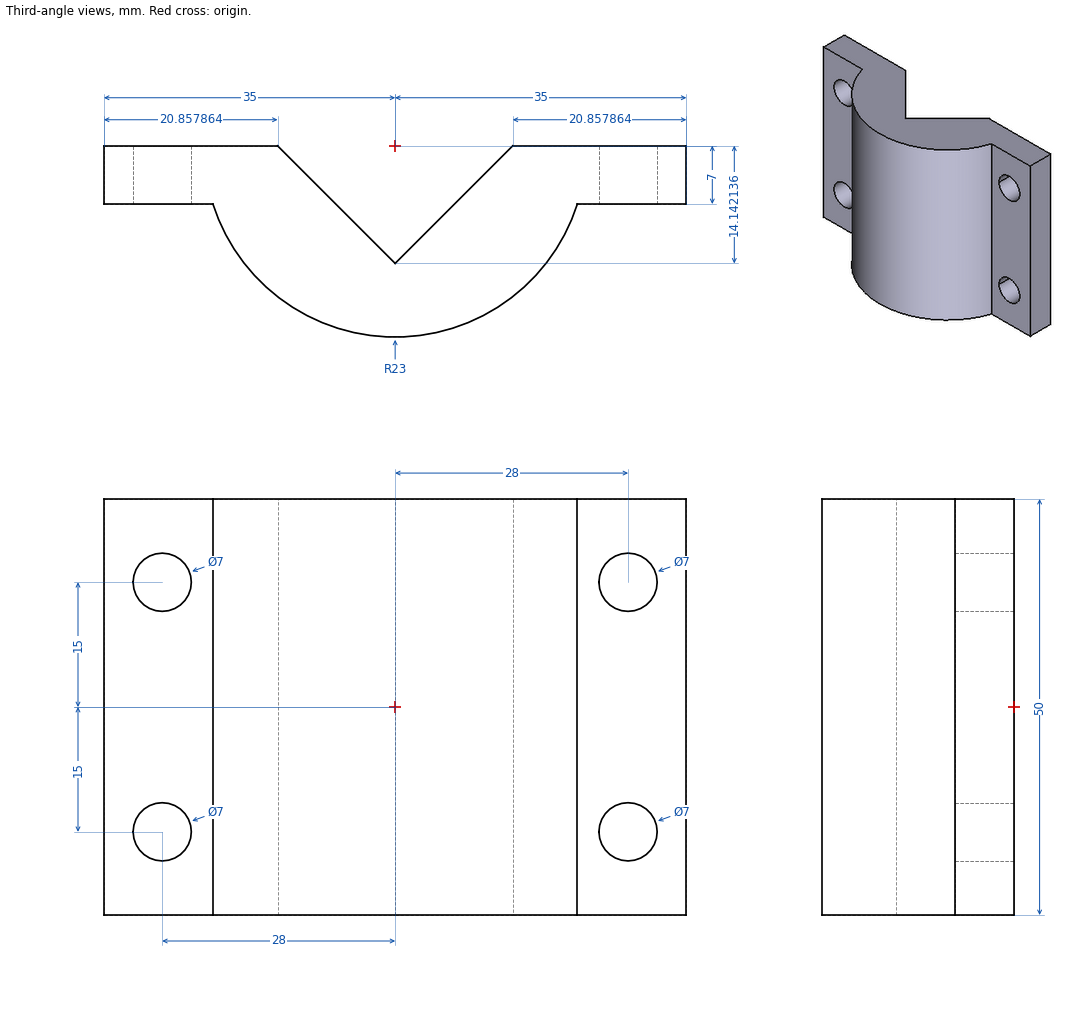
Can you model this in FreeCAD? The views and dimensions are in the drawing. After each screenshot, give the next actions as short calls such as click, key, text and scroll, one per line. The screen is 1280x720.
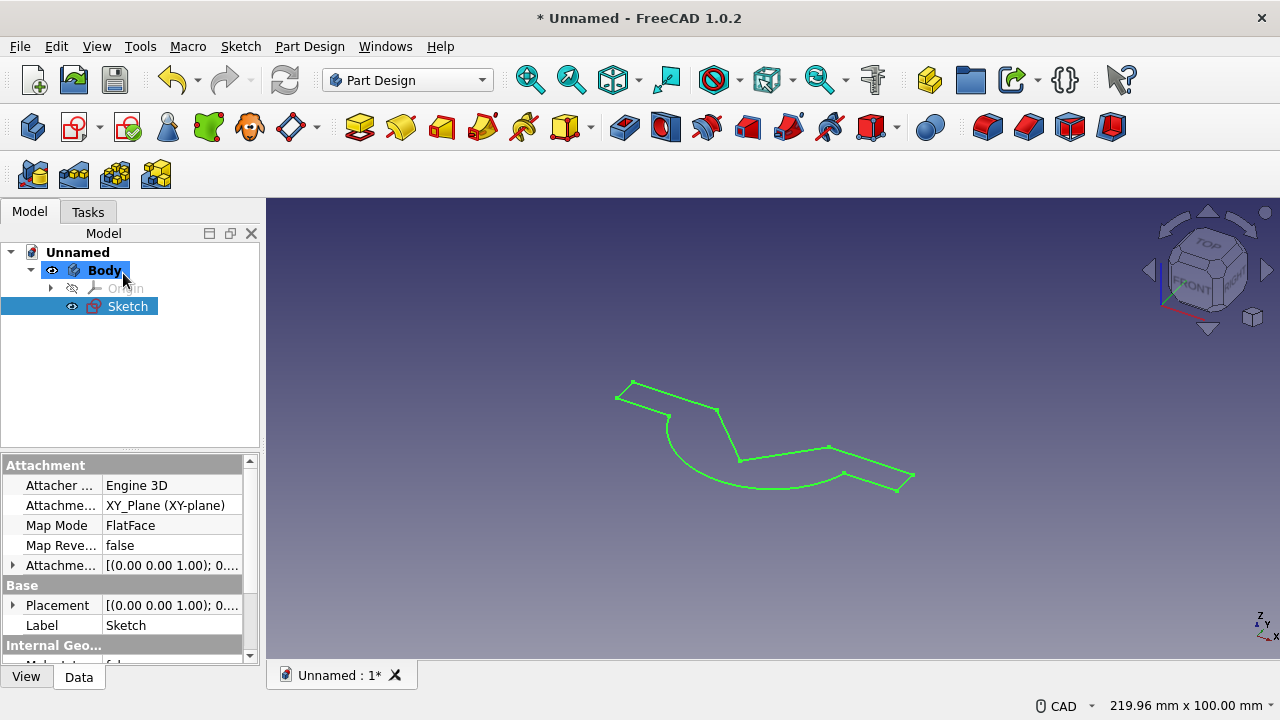
click(360, 128)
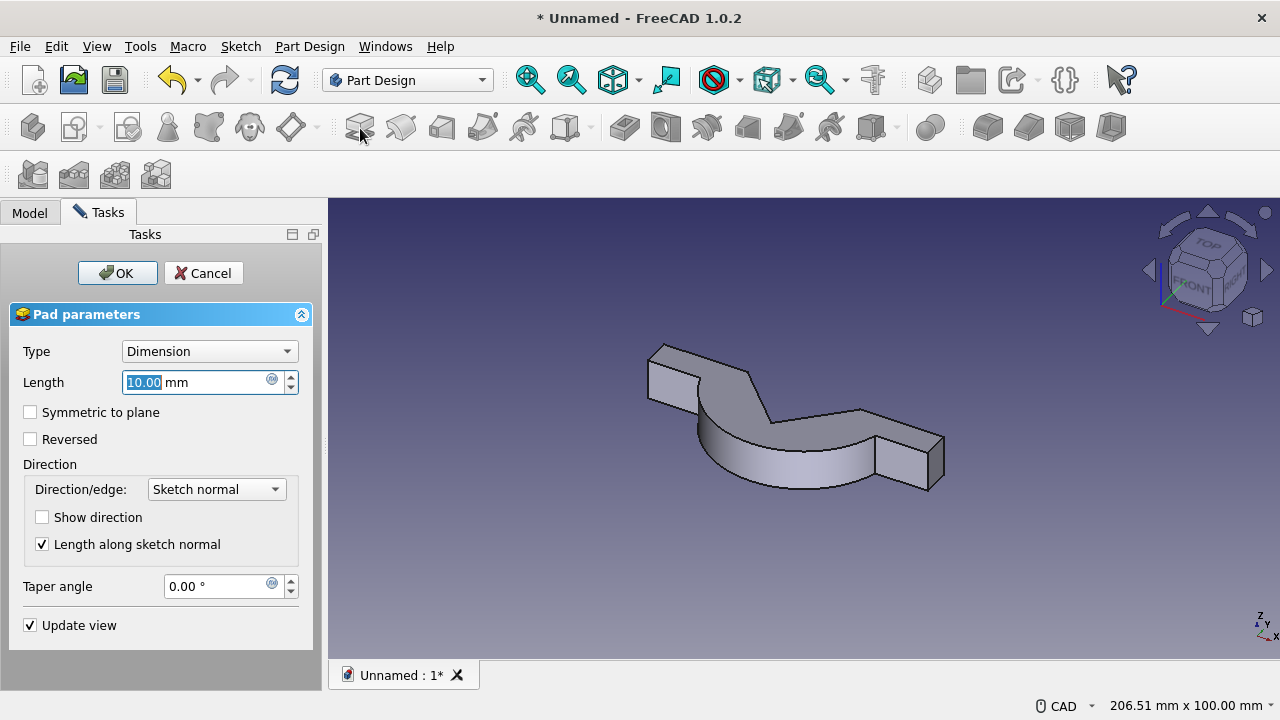
text(50)
key(Tab)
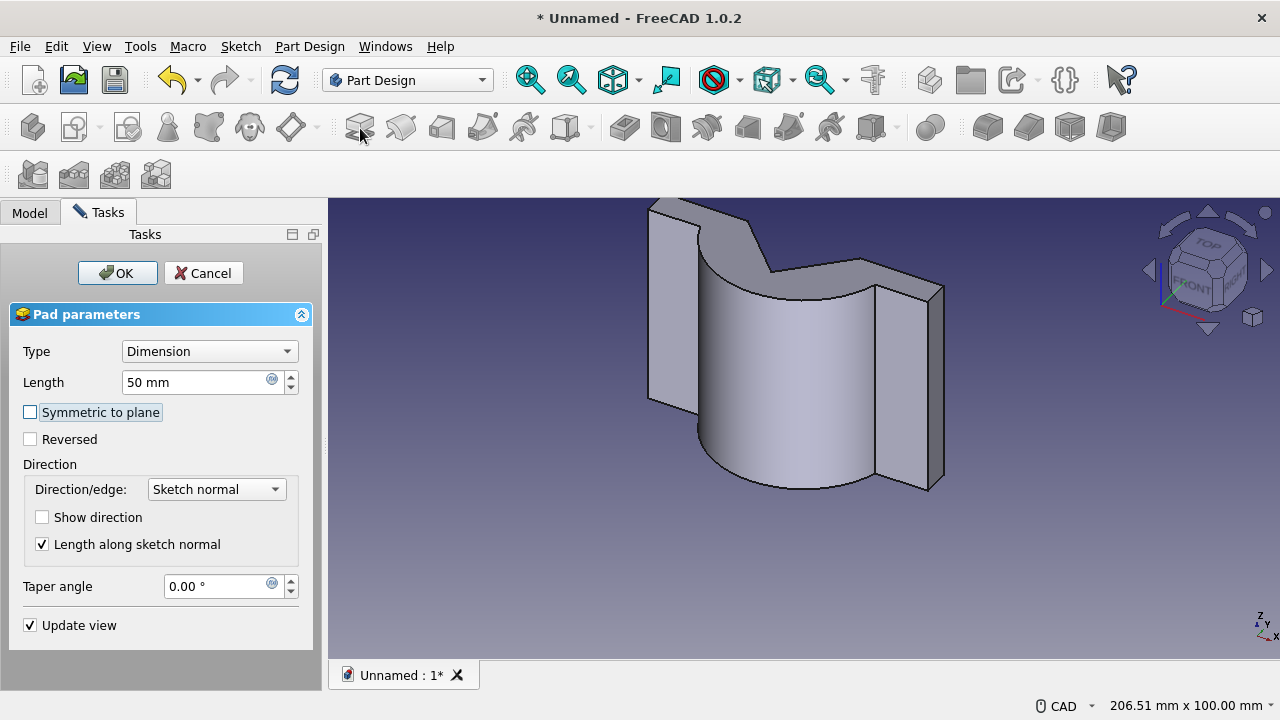
click(31, 412)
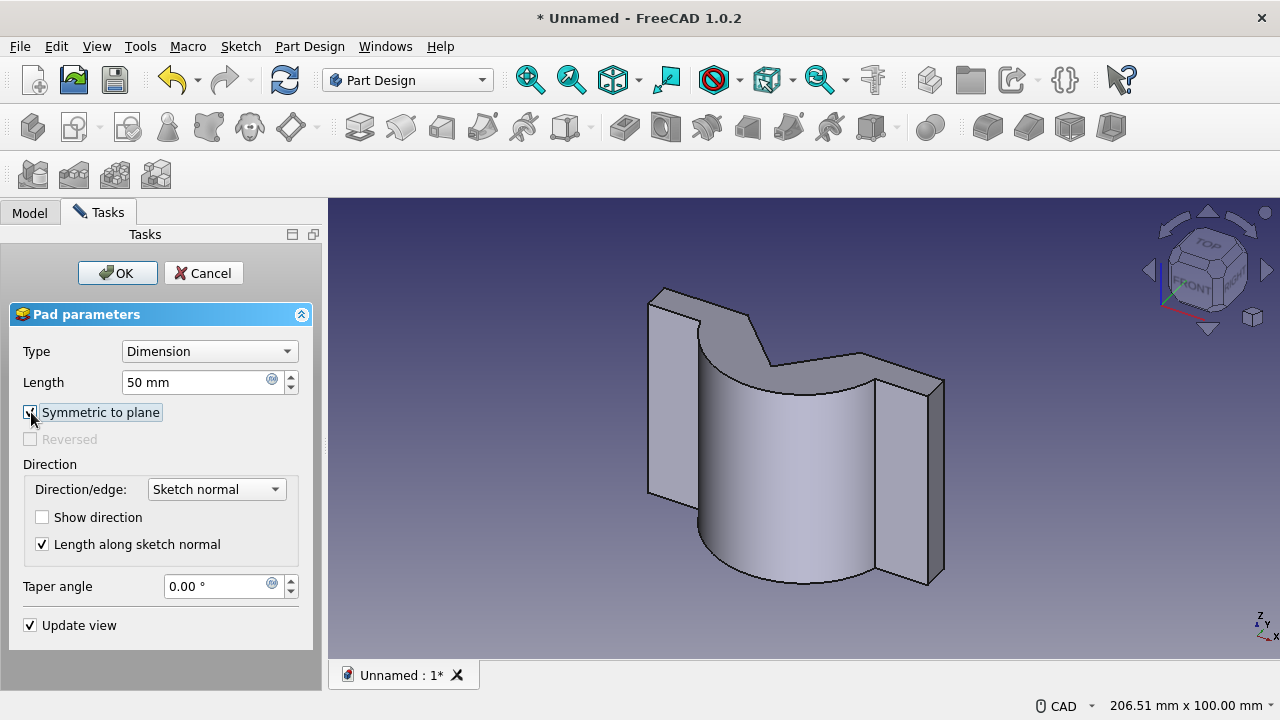
click(118, 273)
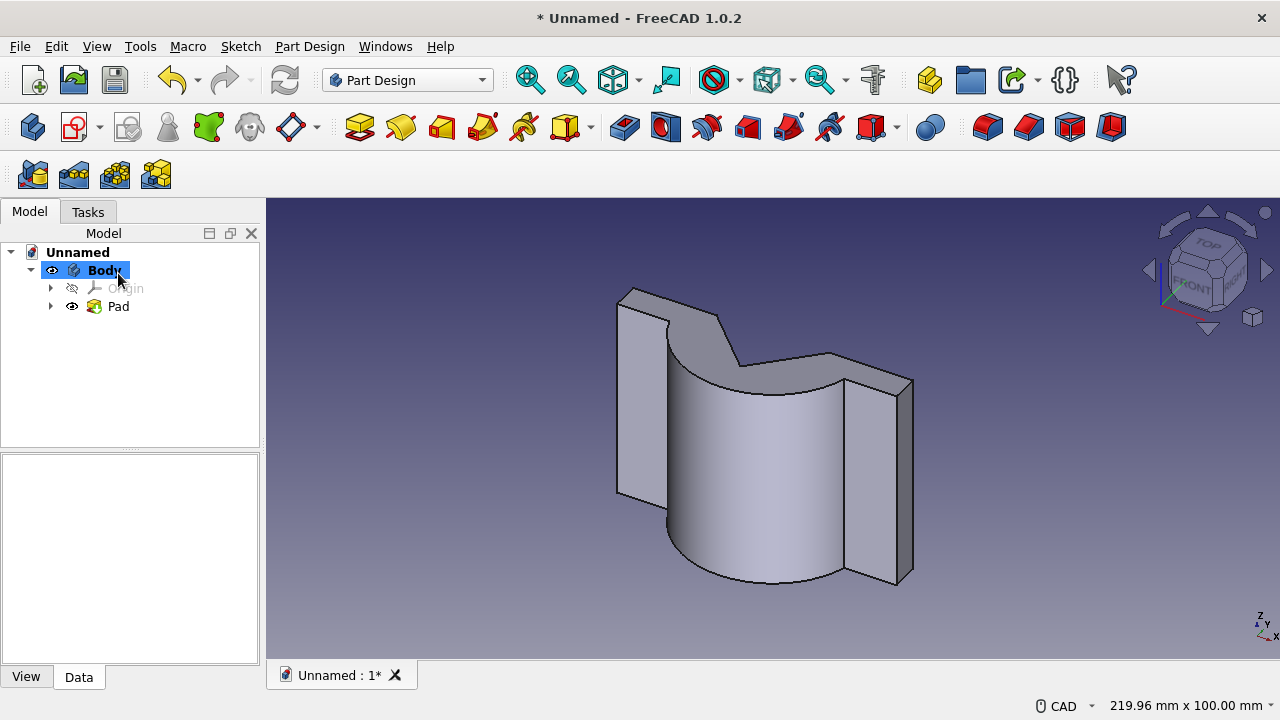
click(74, 128)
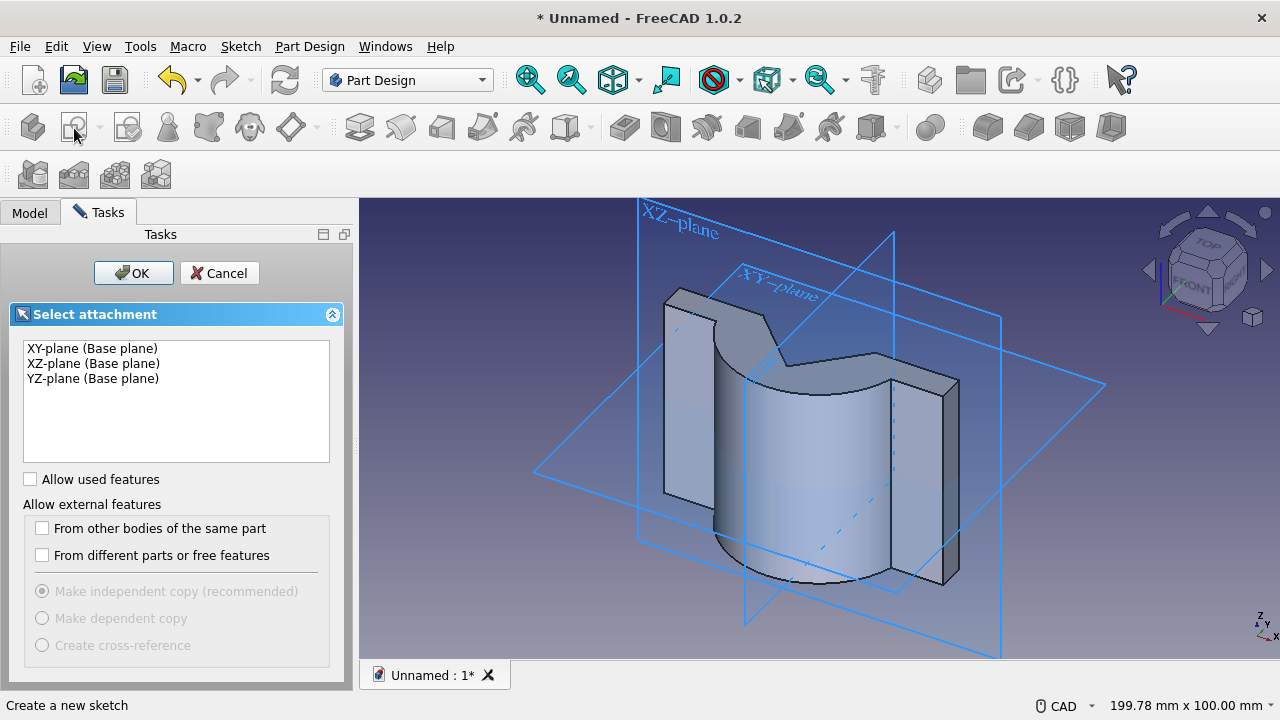
click(84, 364)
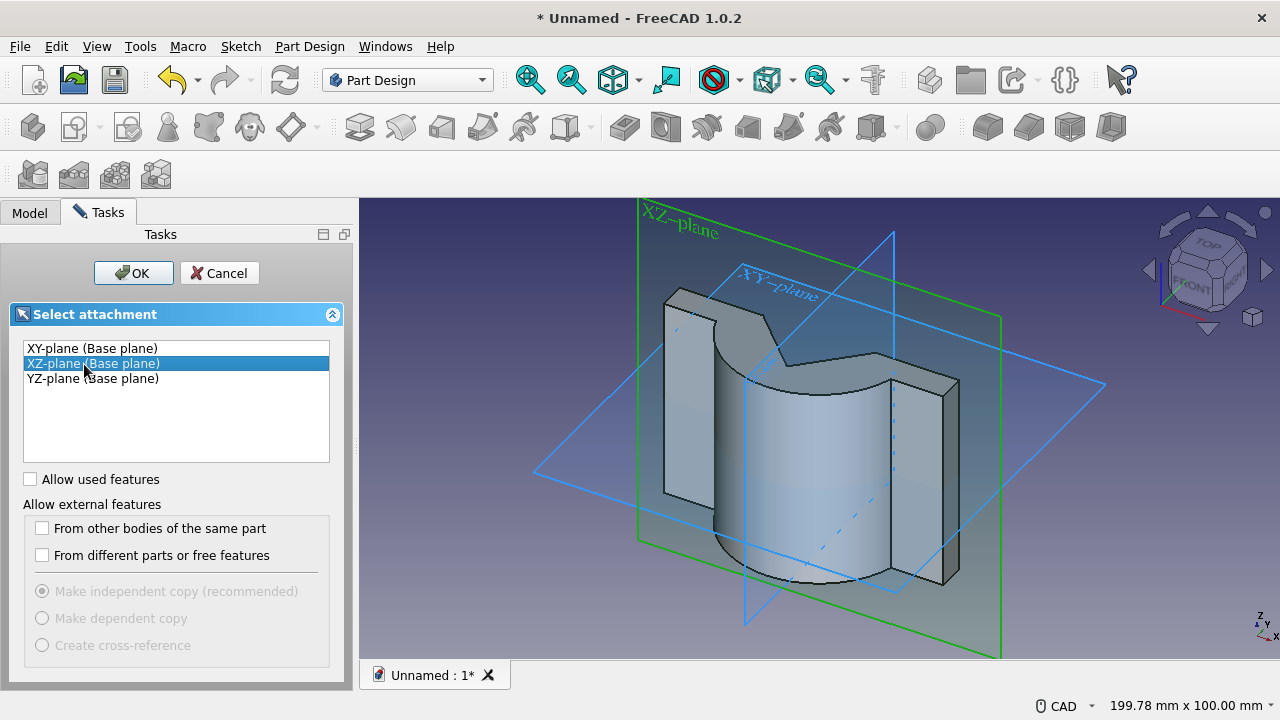
click(134, 273)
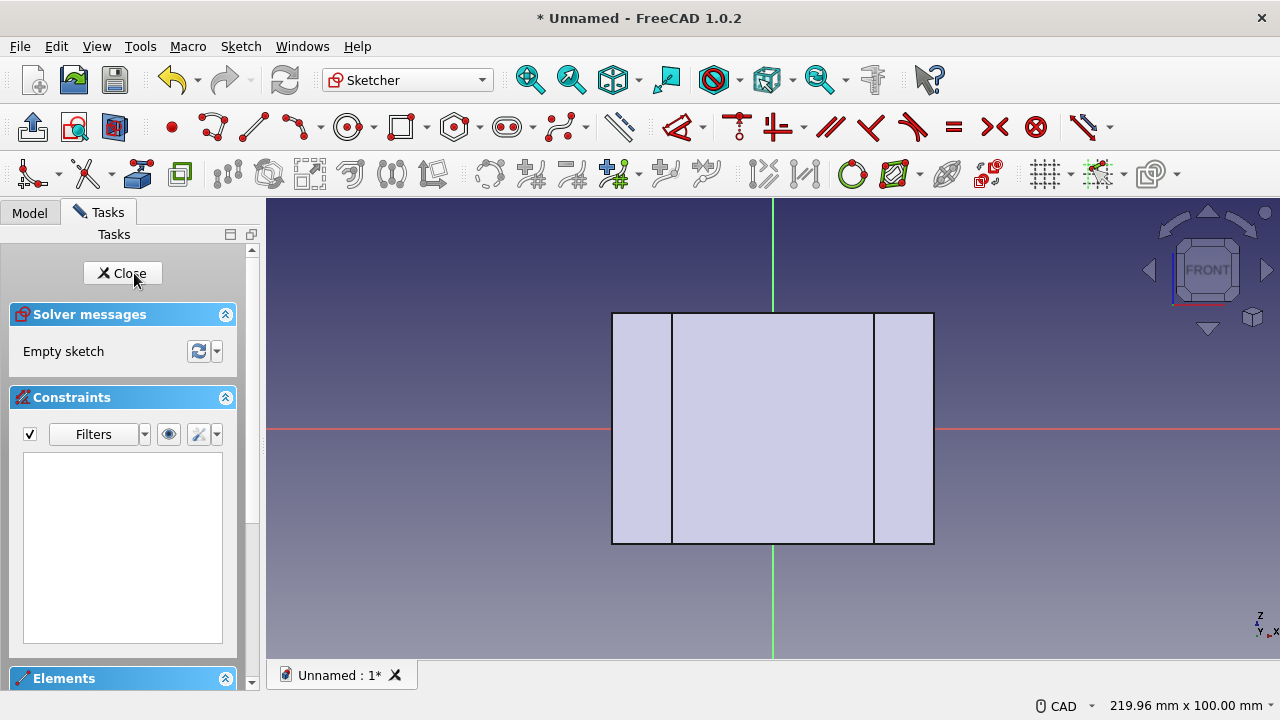
key(q)
key(s)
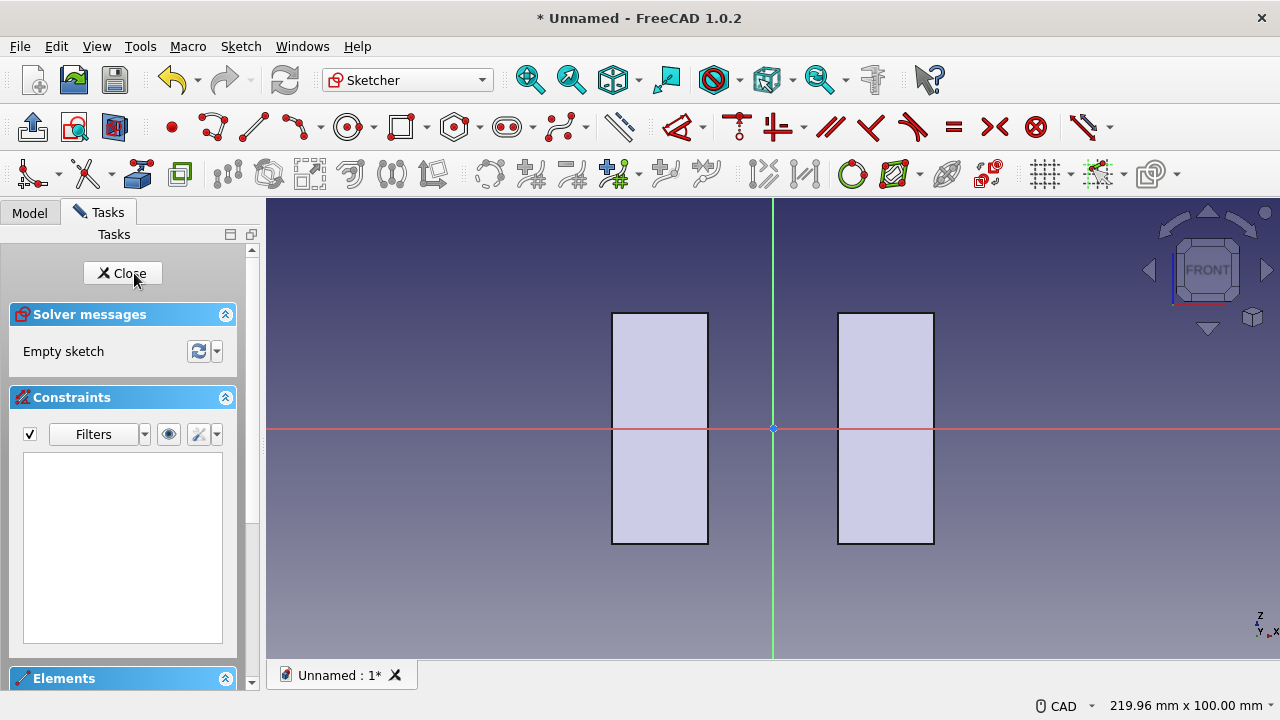
scroll(636, 506, up, 11)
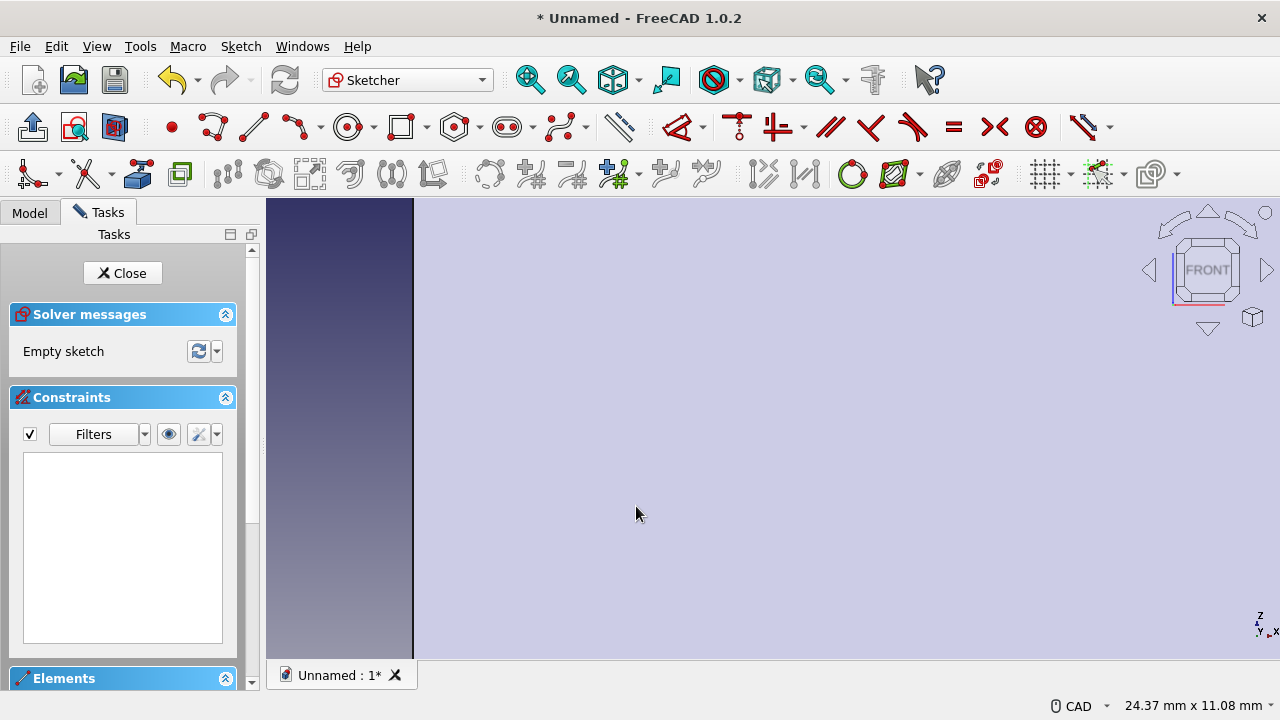
key(g)
key(c)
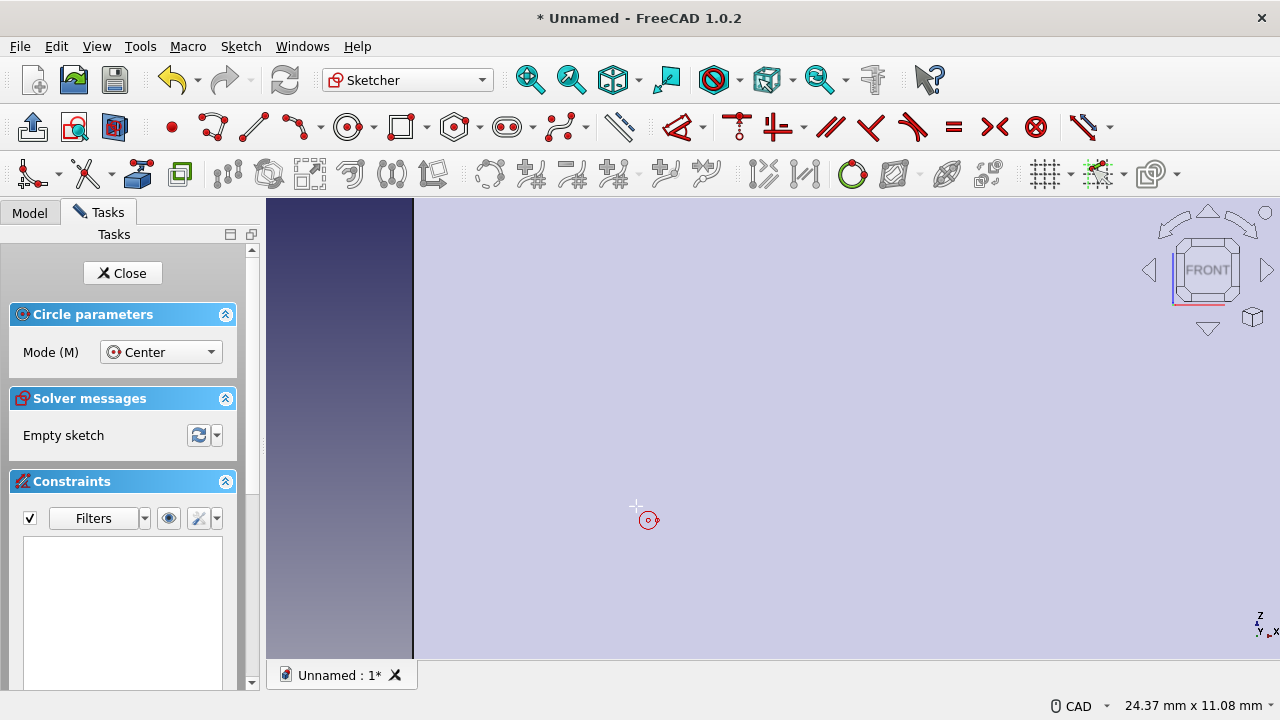
click(705, 425)
click(808, 322)
key(Escape)